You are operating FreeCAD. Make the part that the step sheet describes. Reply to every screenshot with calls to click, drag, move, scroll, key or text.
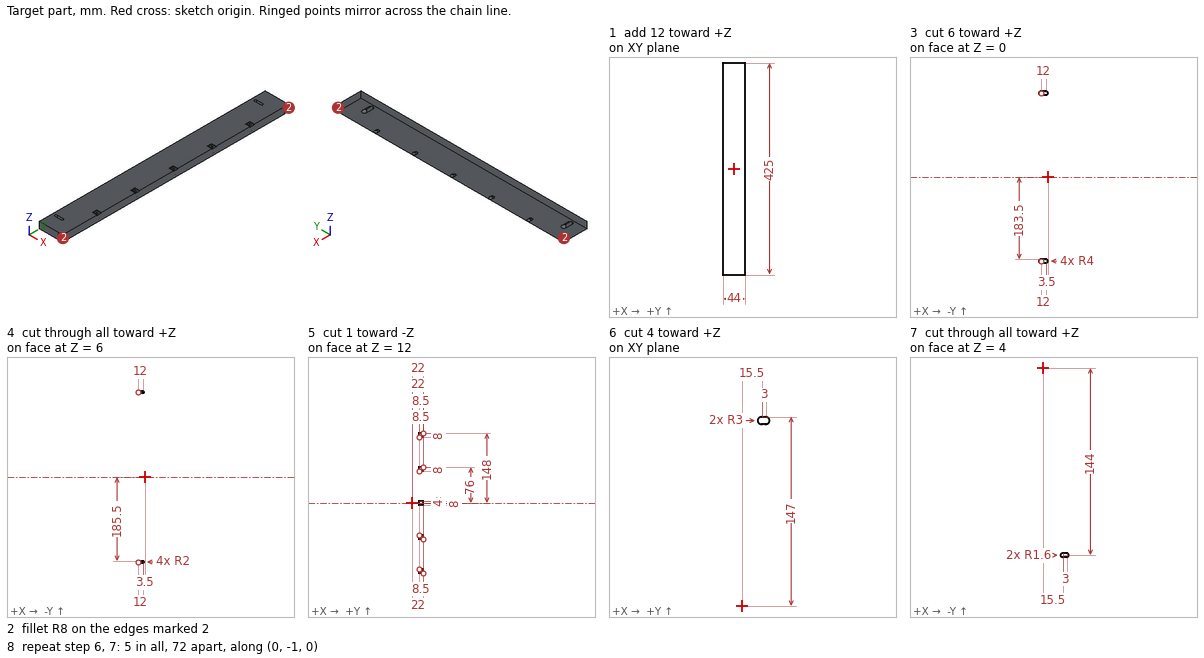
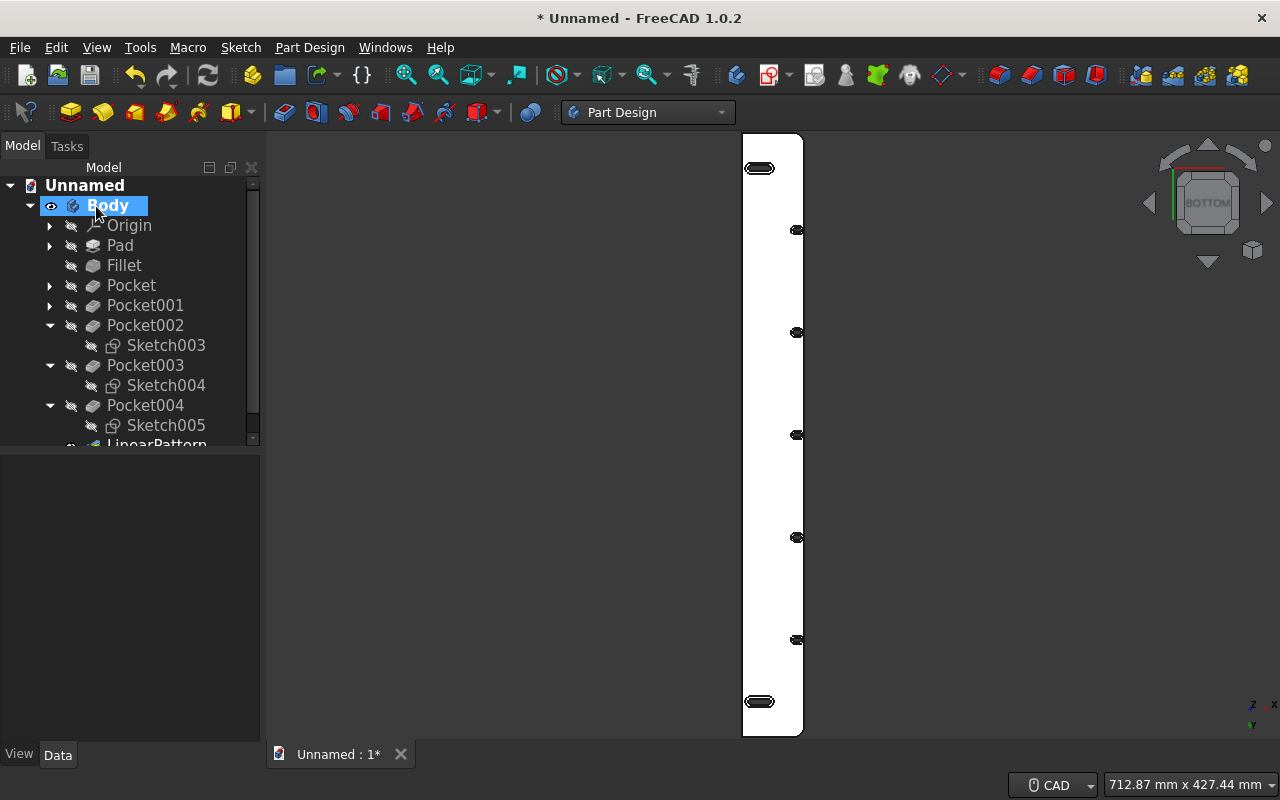
key(0)